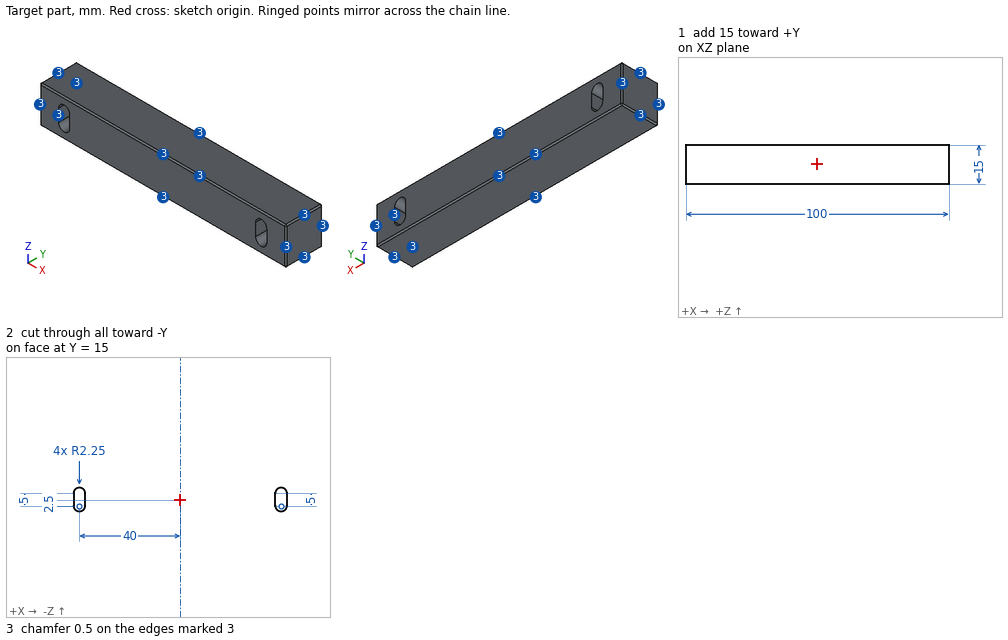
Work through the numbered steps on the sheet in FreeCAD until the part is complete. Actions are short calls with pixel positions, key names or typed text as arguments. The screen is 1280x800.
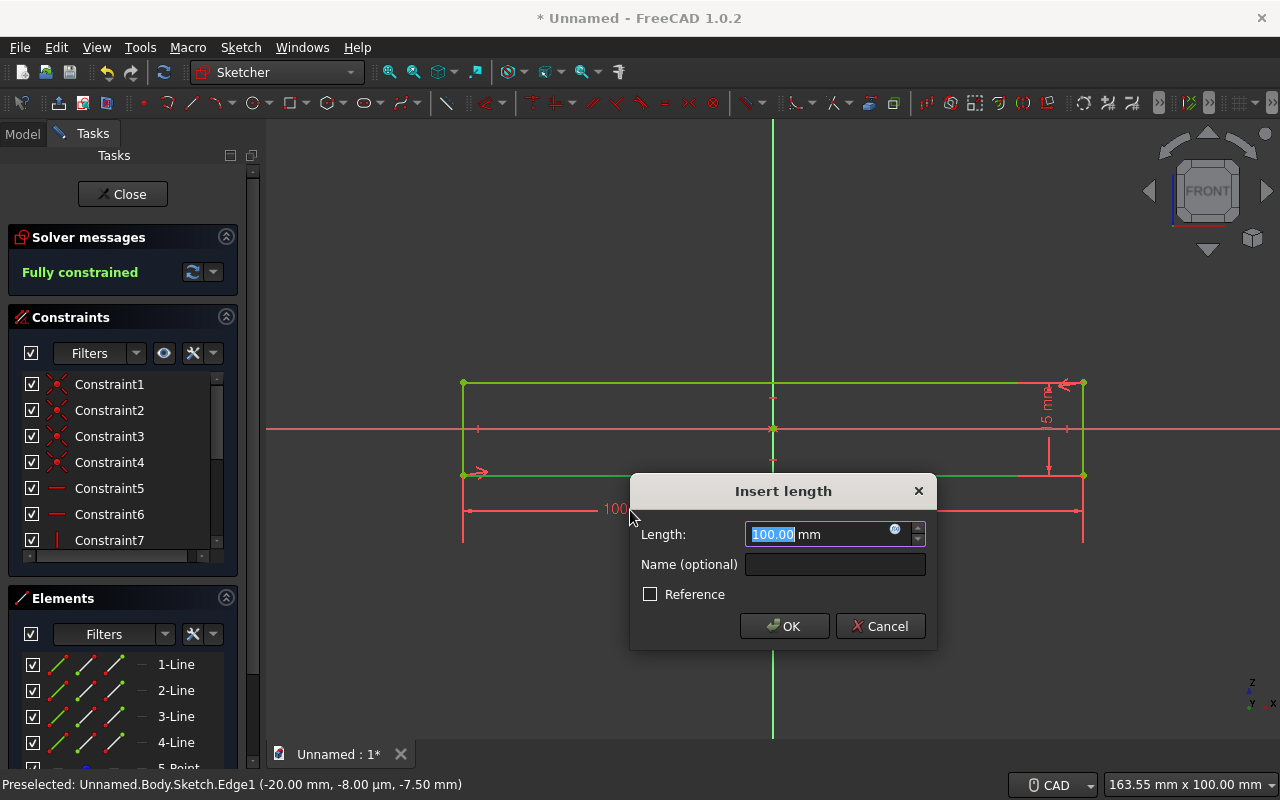
text(100)
key(Return)
key(Escape)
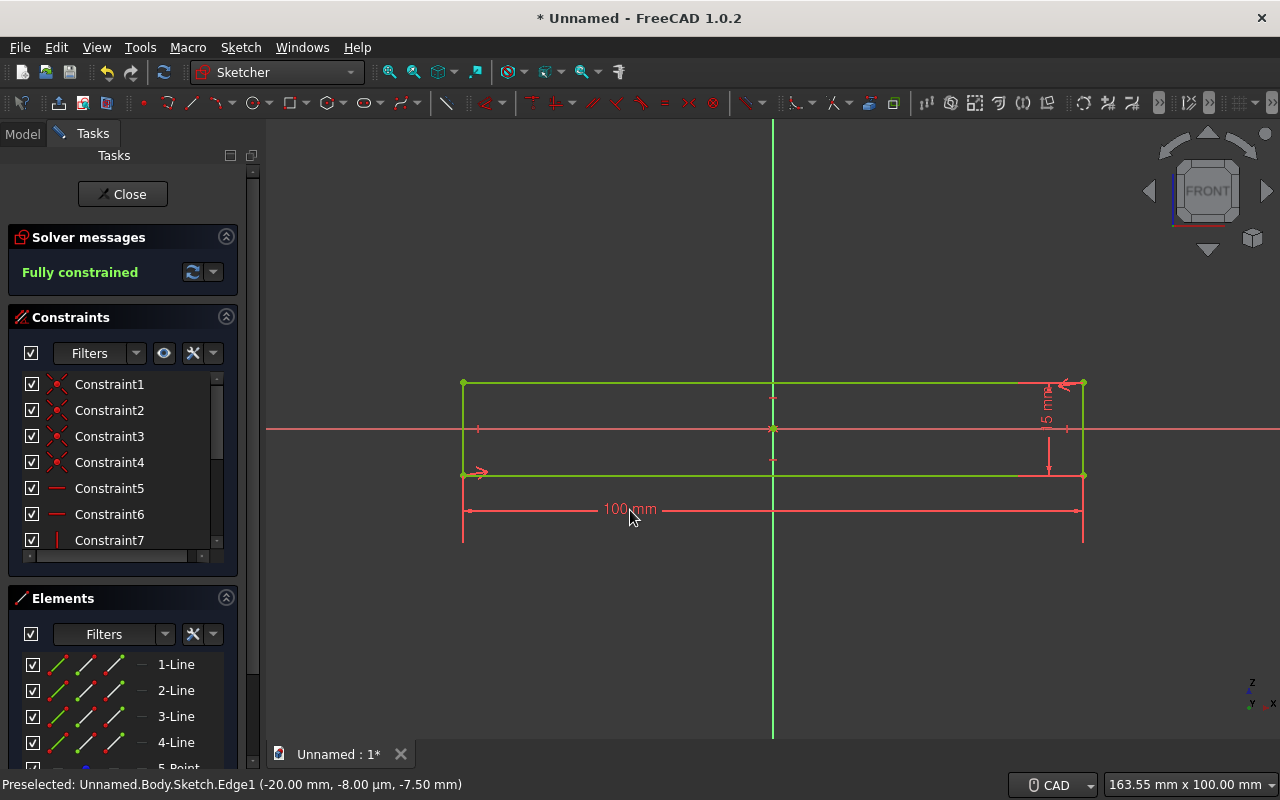
click(123, 194)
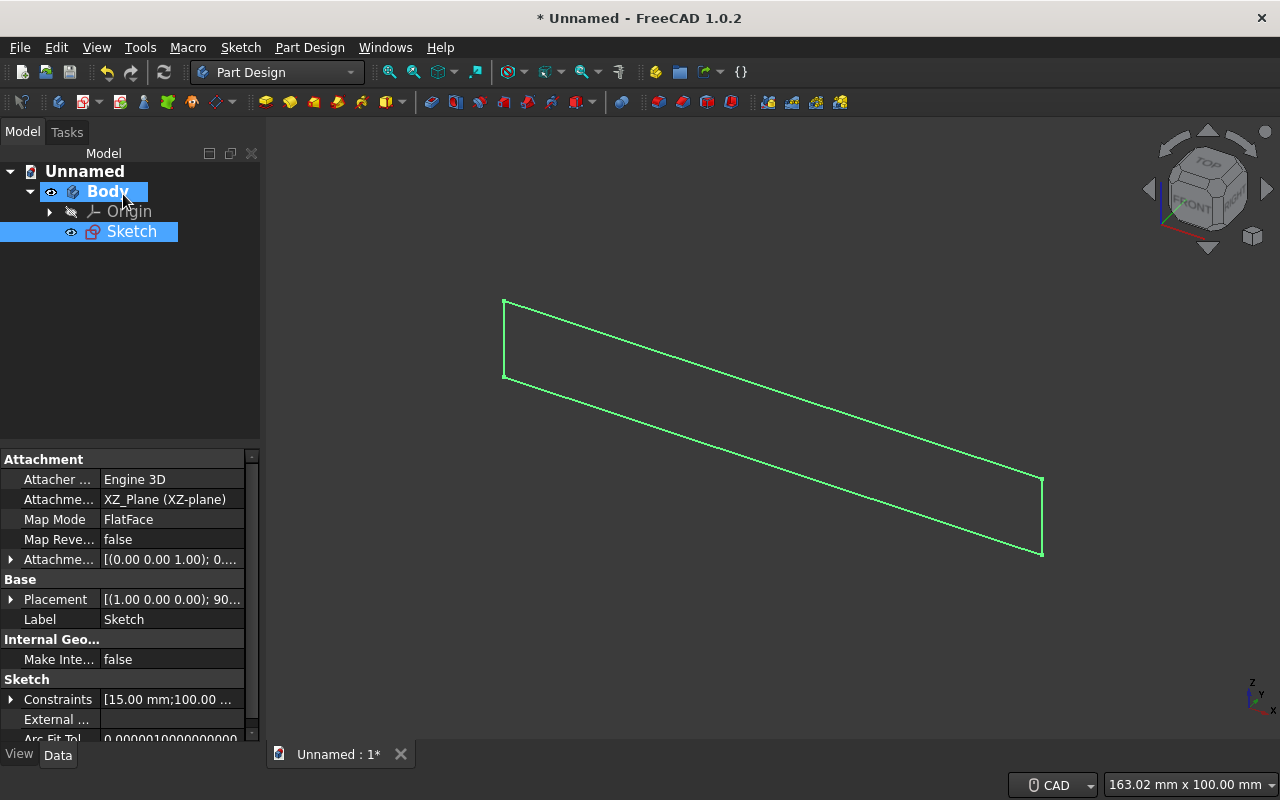
click(266, 102)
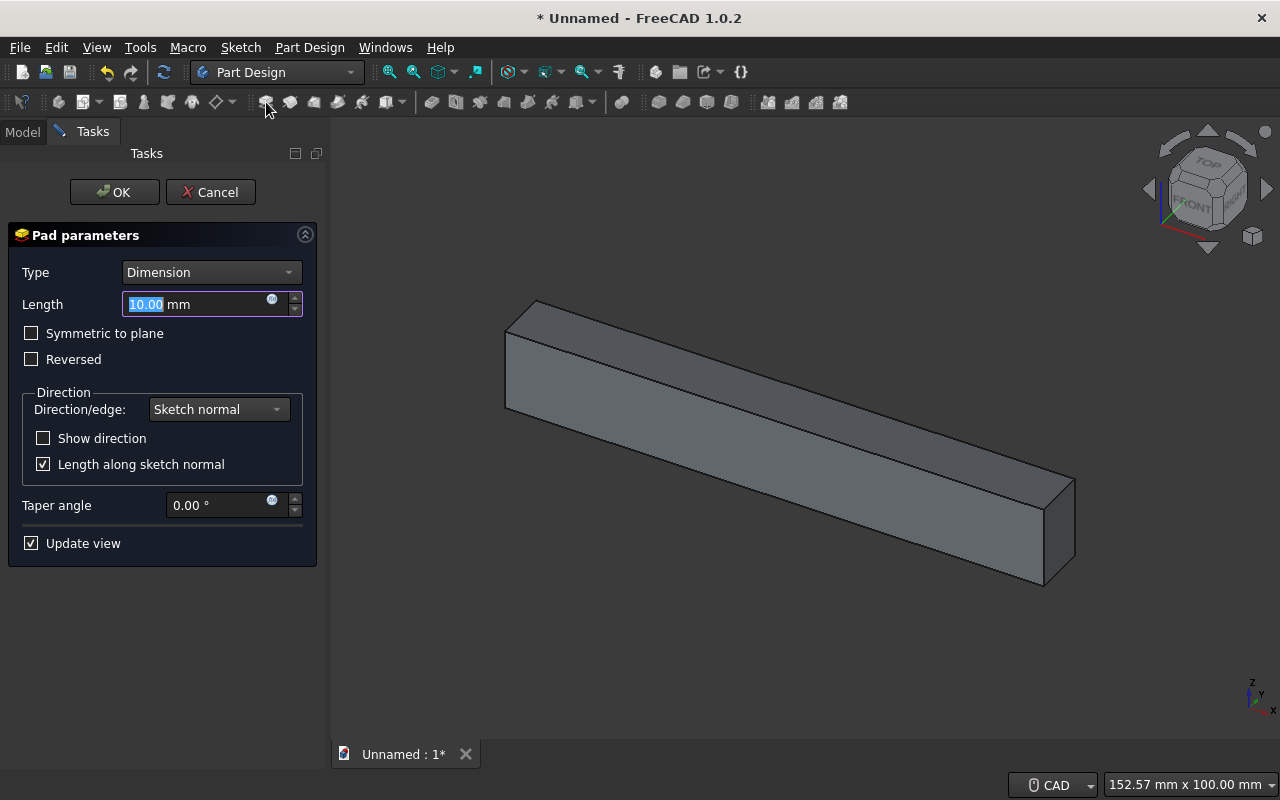
text(15)
key(Tab)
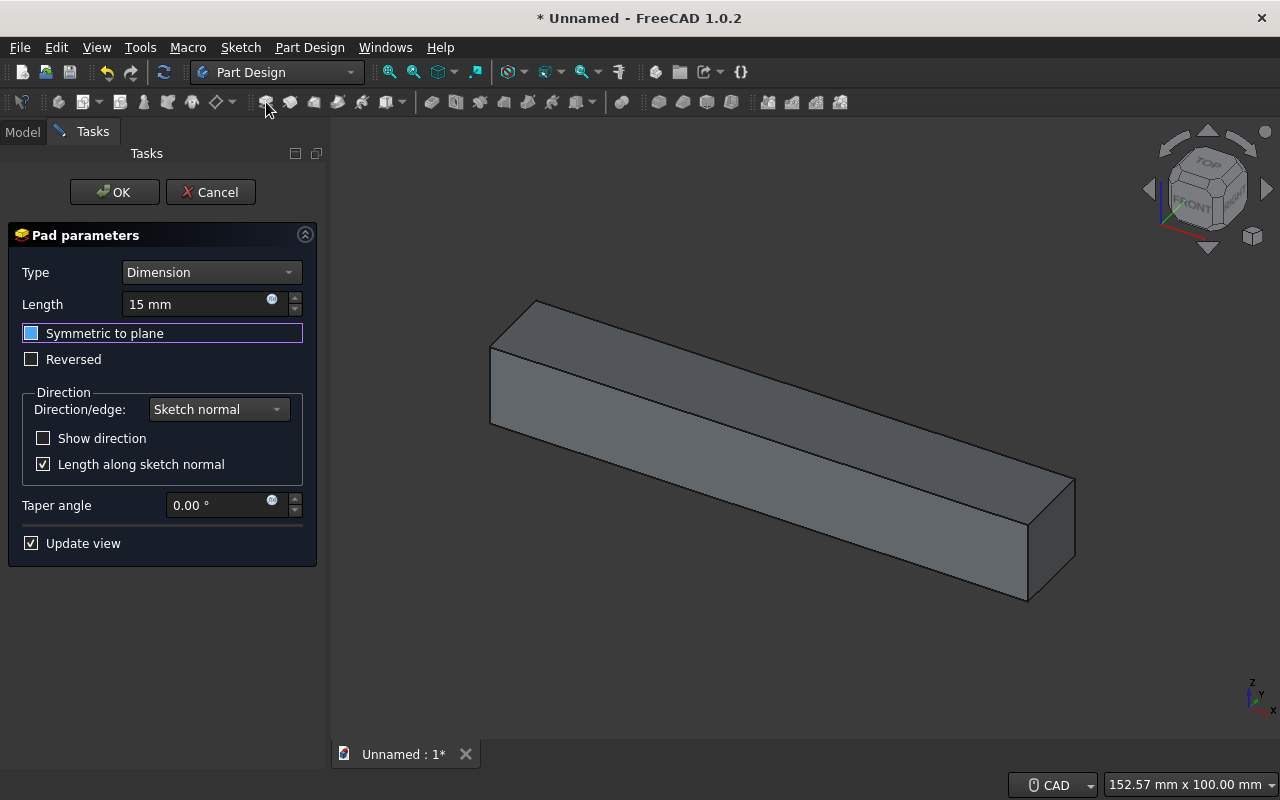
click(30, 359)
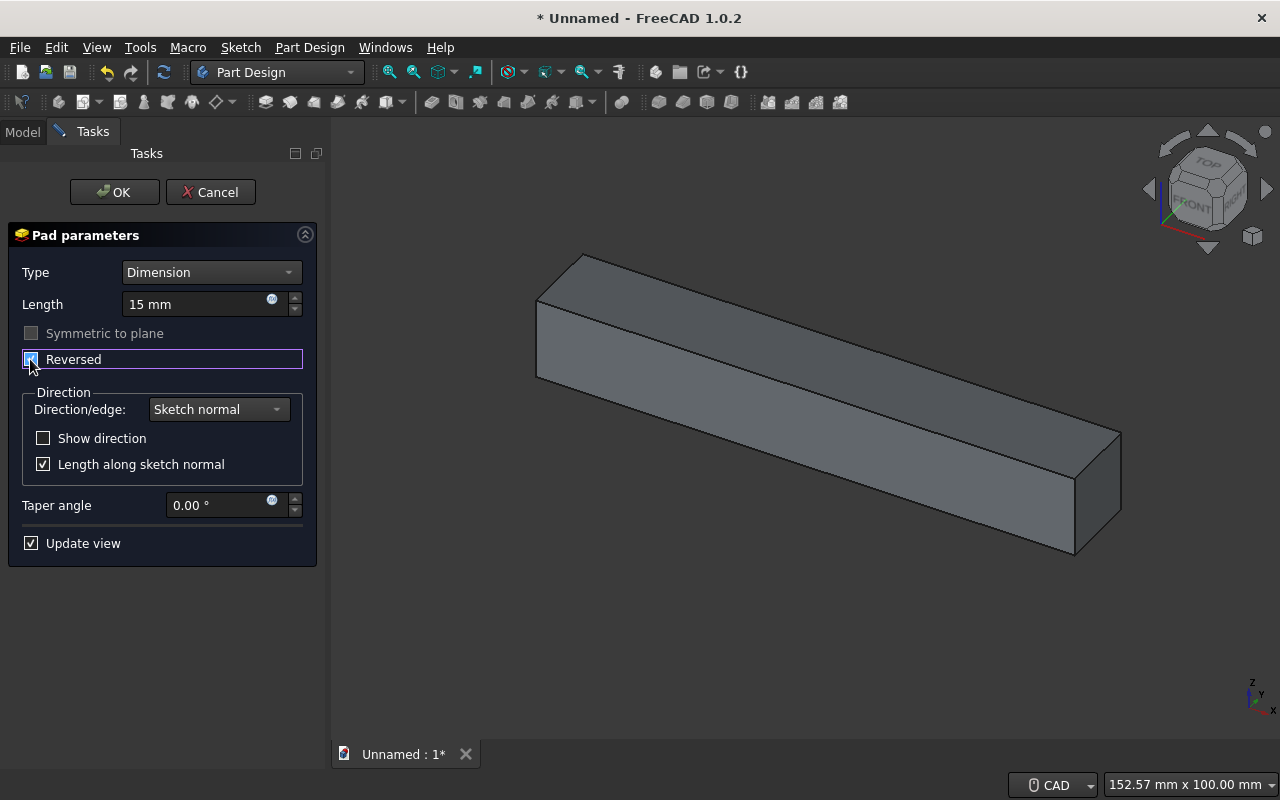
click(115, 192)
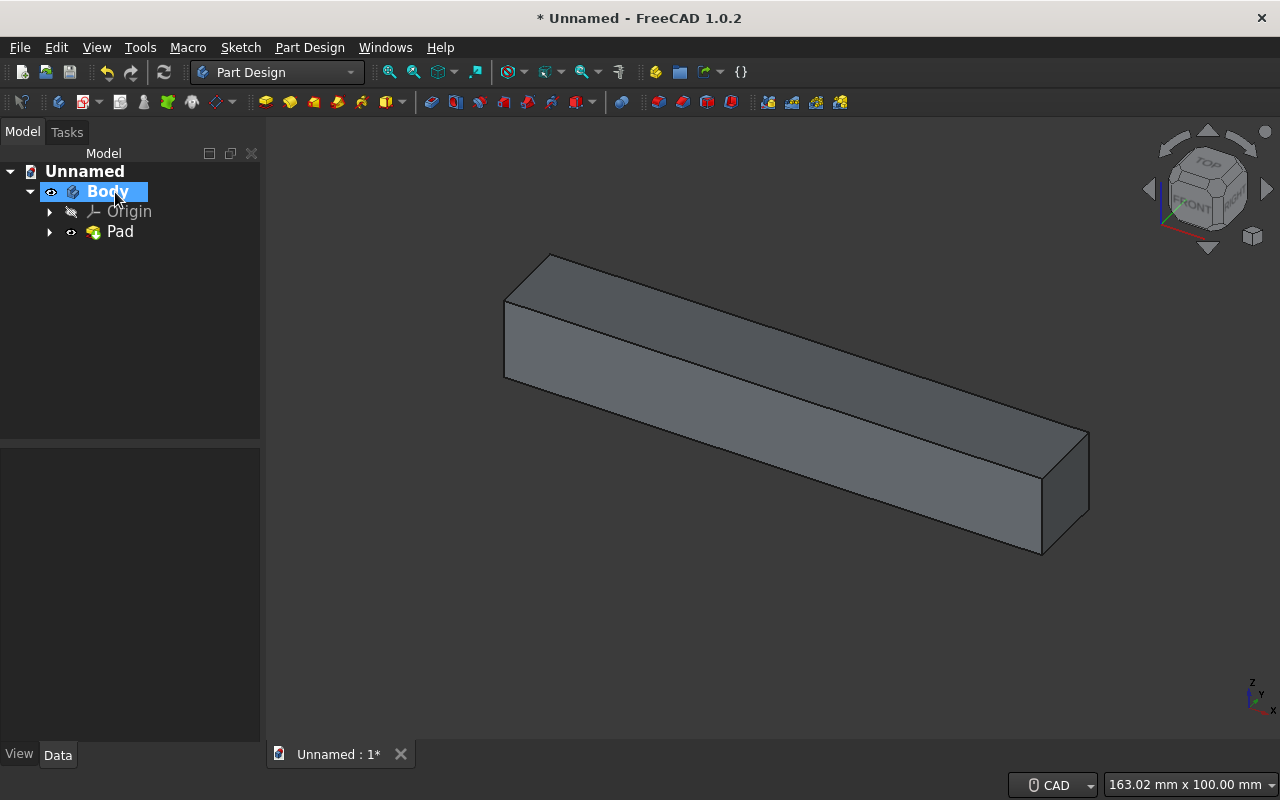
key(4)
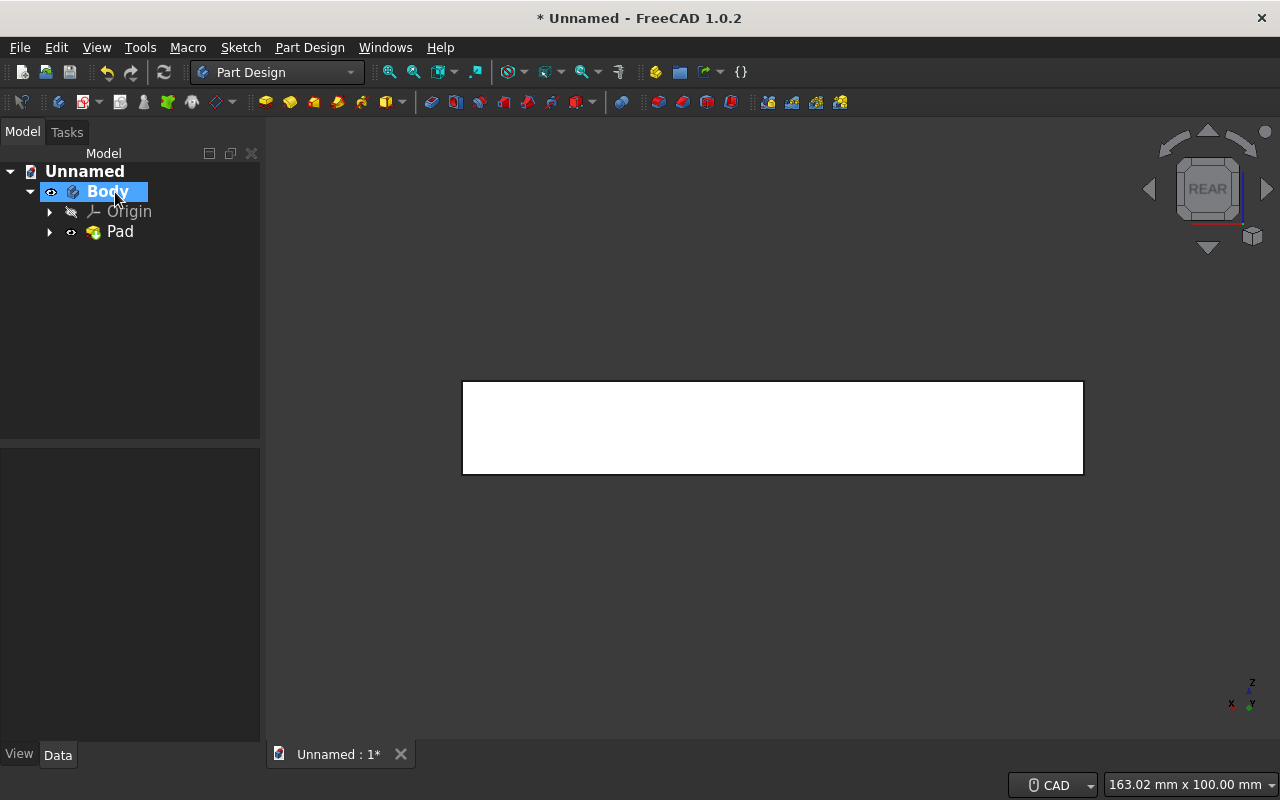
click(595, 427)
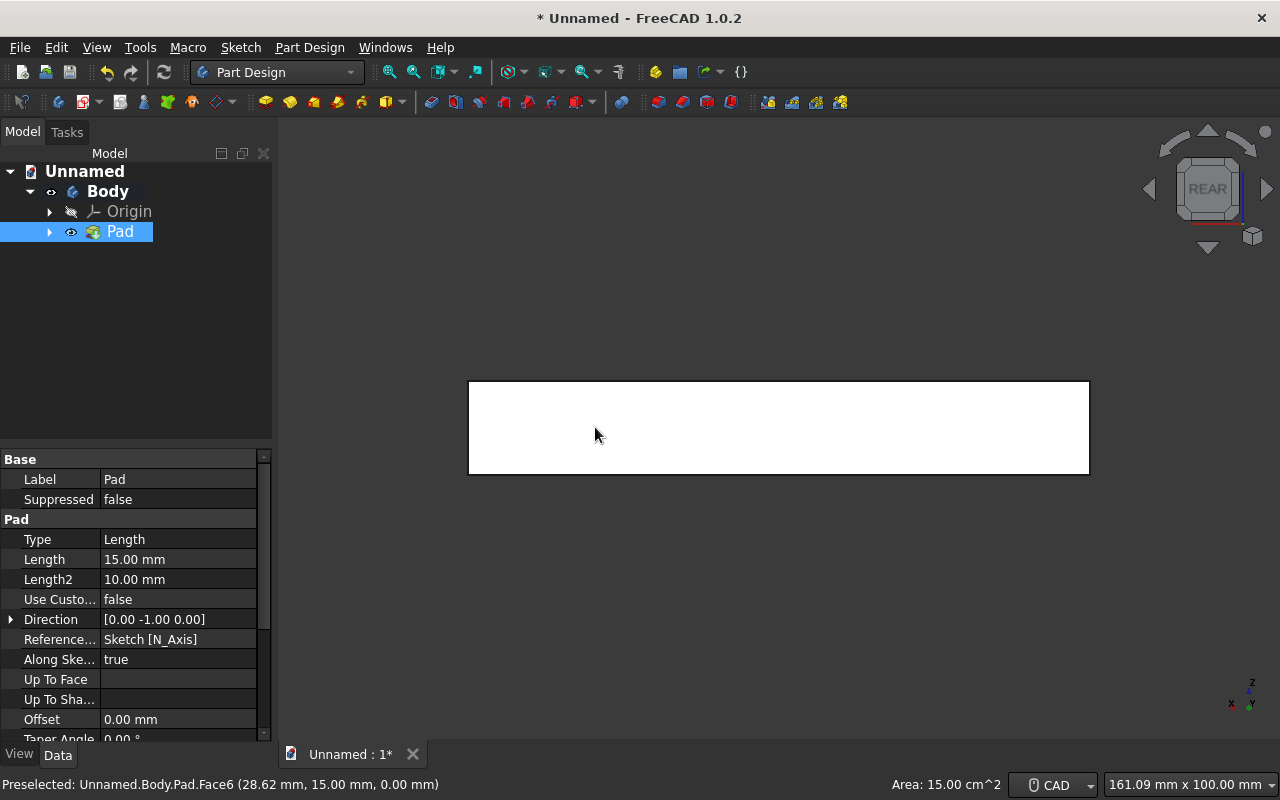
click(84, 102)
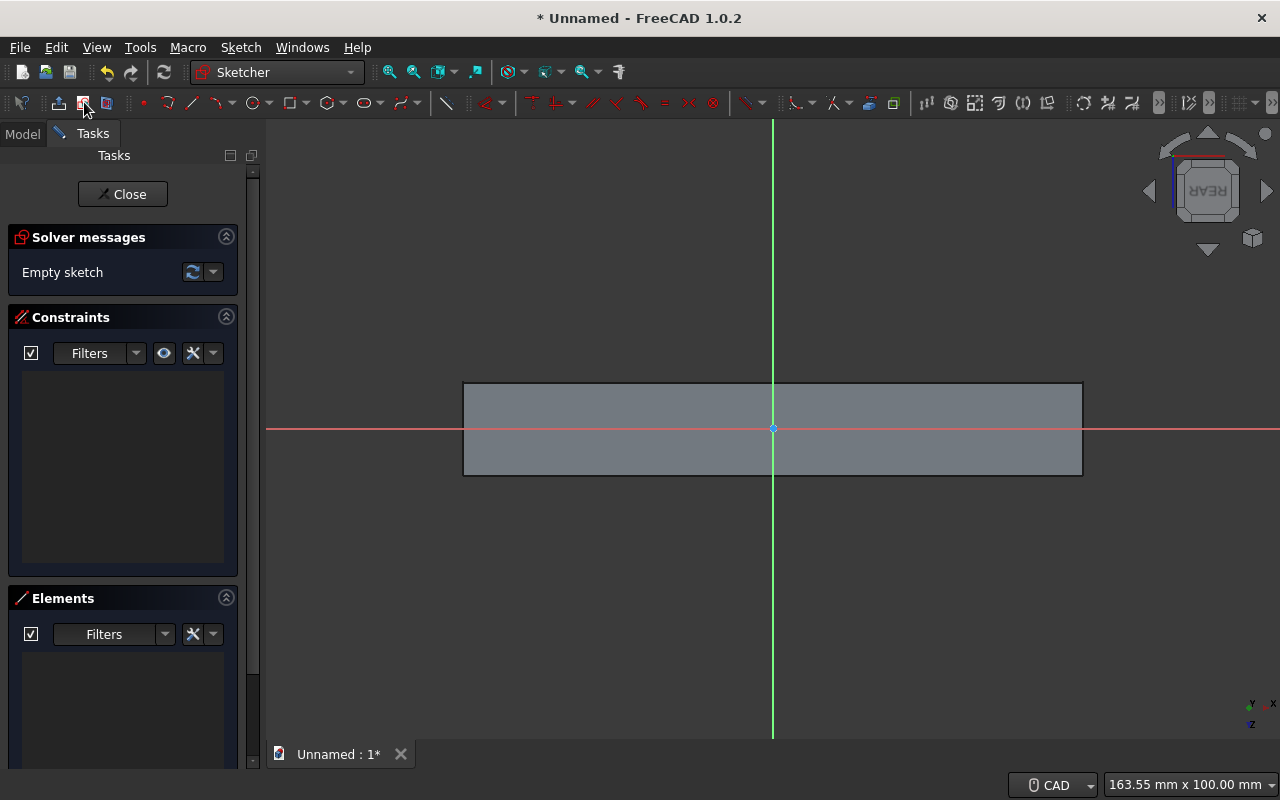
click(364, 104)